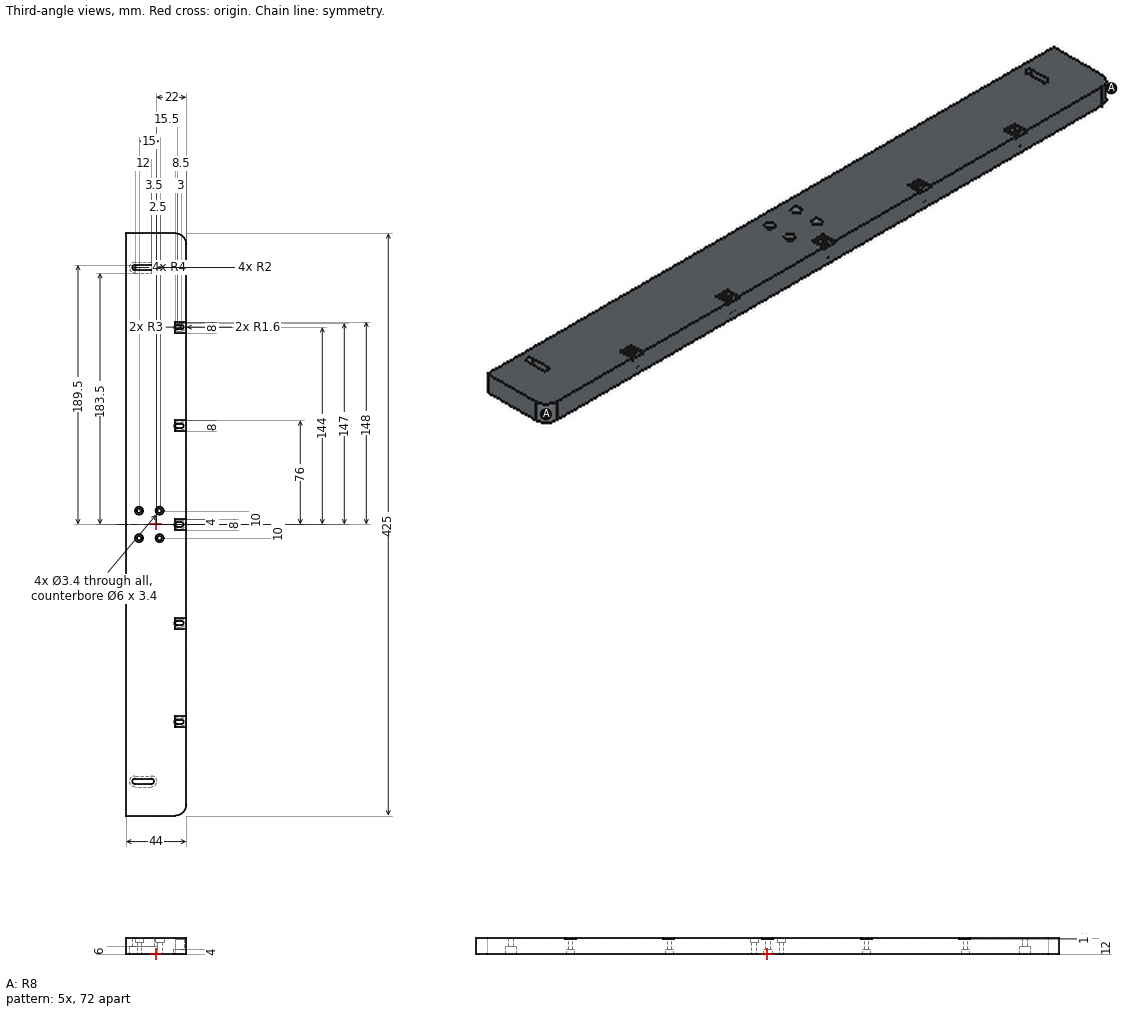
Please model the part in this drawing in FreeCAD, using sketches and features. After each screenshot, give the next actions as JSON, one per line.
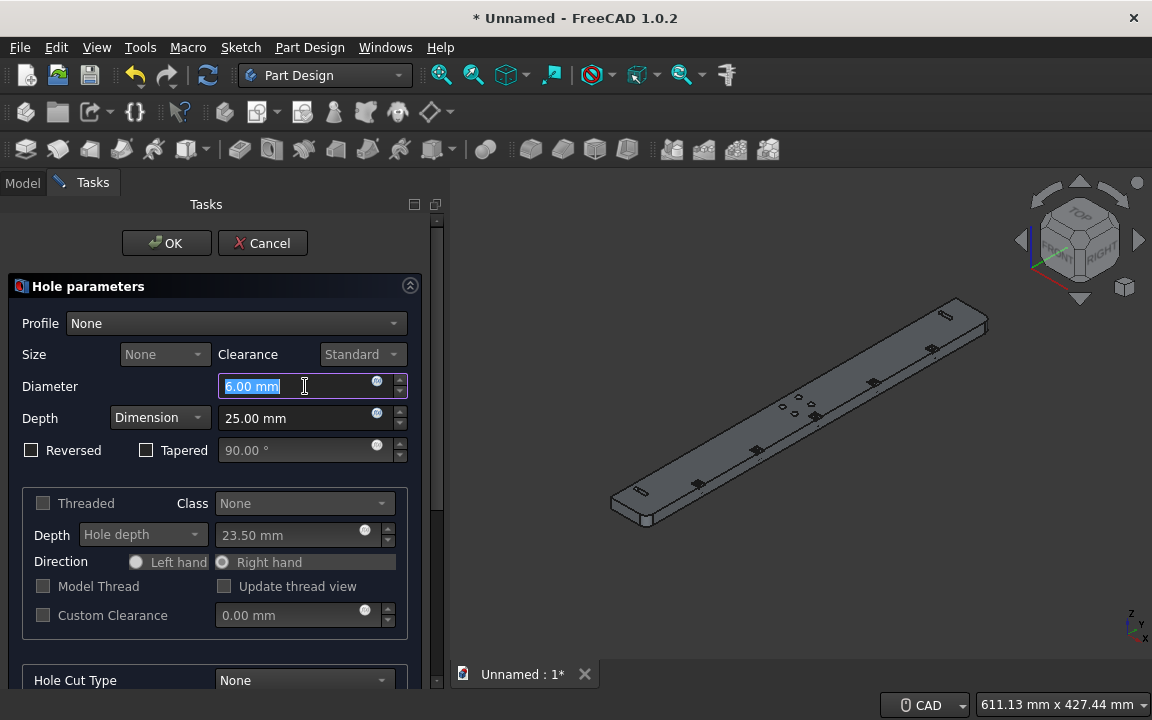
{"action": "type", "text": "3.4"}
{"action": "key", "text": "Tab"}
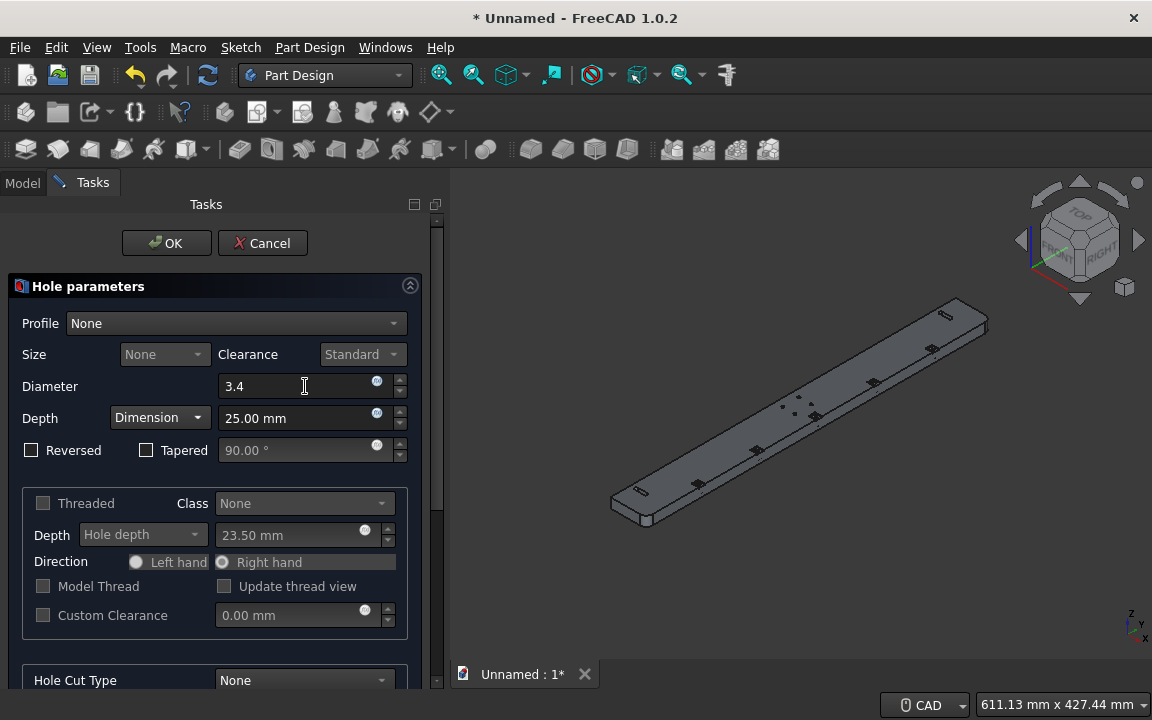
{"action": "left_click", "coordinate": [161, 418]}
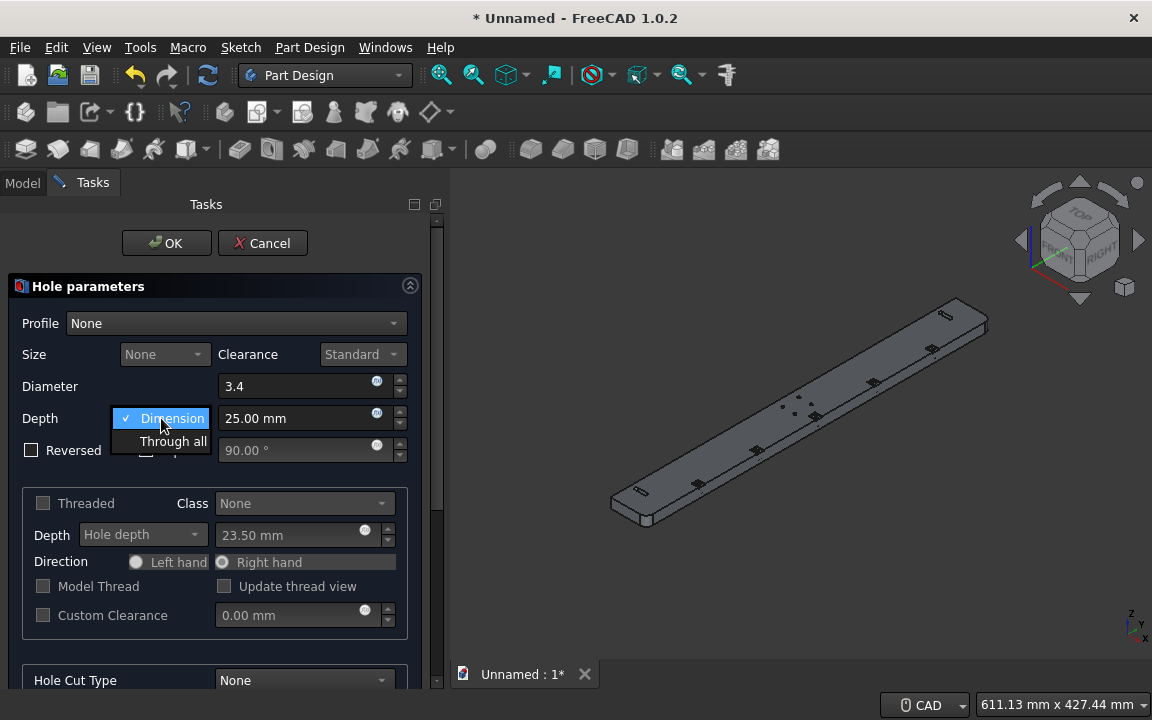
{"action": "left_click", "coordinate": [160, 442]}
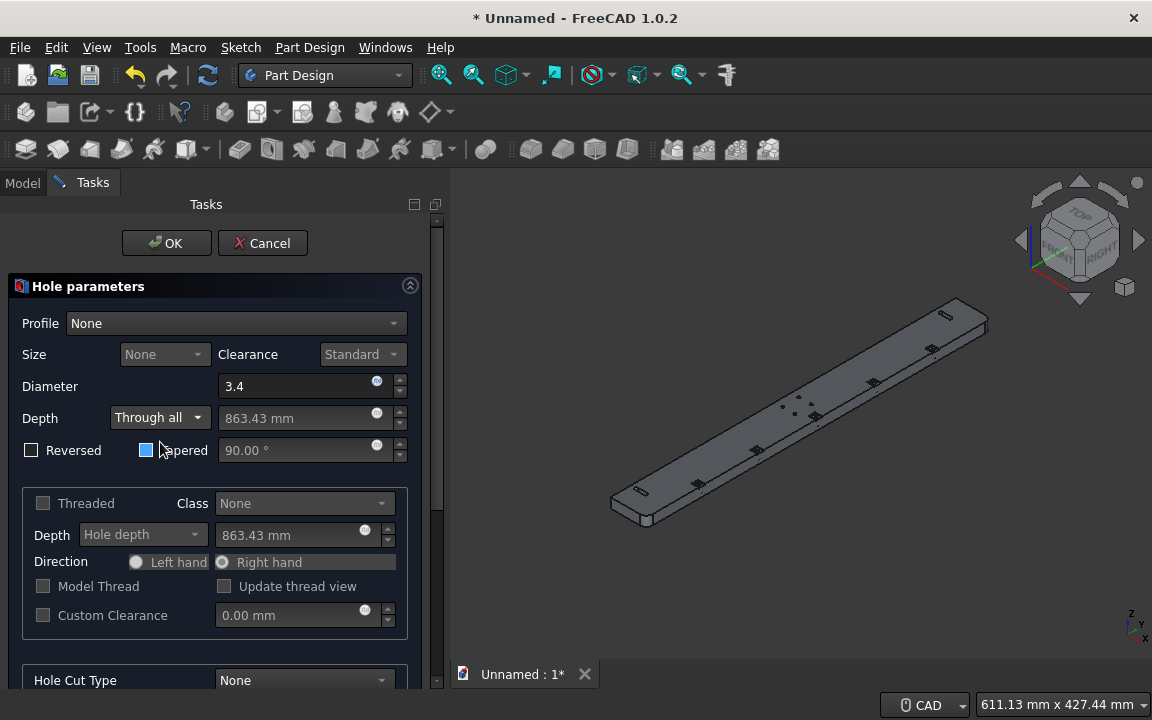
{"action": "scroll", "coordinate": [437, 451], "scroll_direction": "down", "scroll_amount": 2}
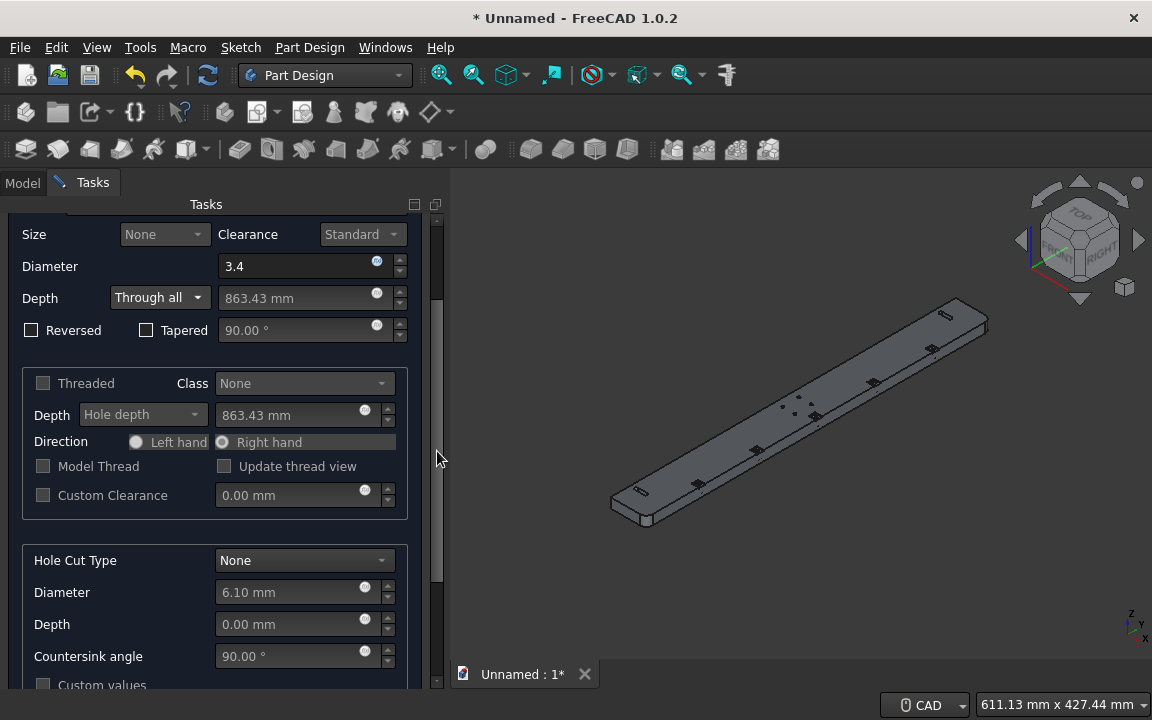
{"action": "left_click", "coordinate": [306, 560]}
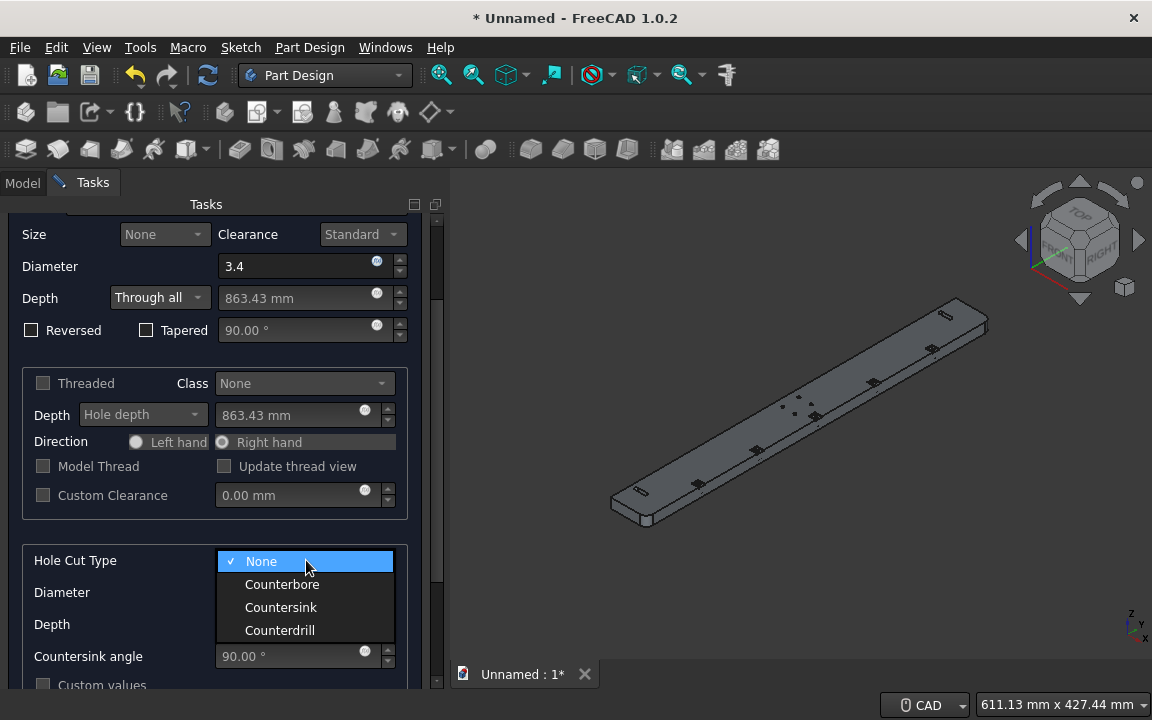
{"action": "left_click", "coordinate": [304, 584]}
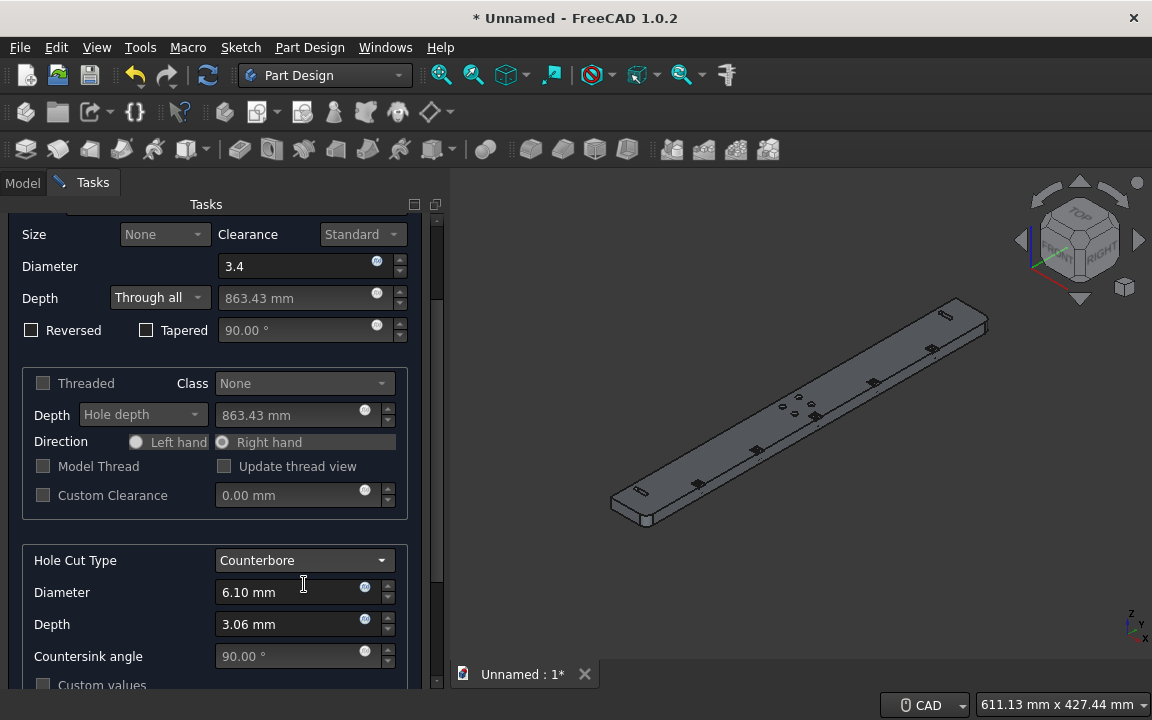
{"action": "triple_click", "coordinate": [298, 592]}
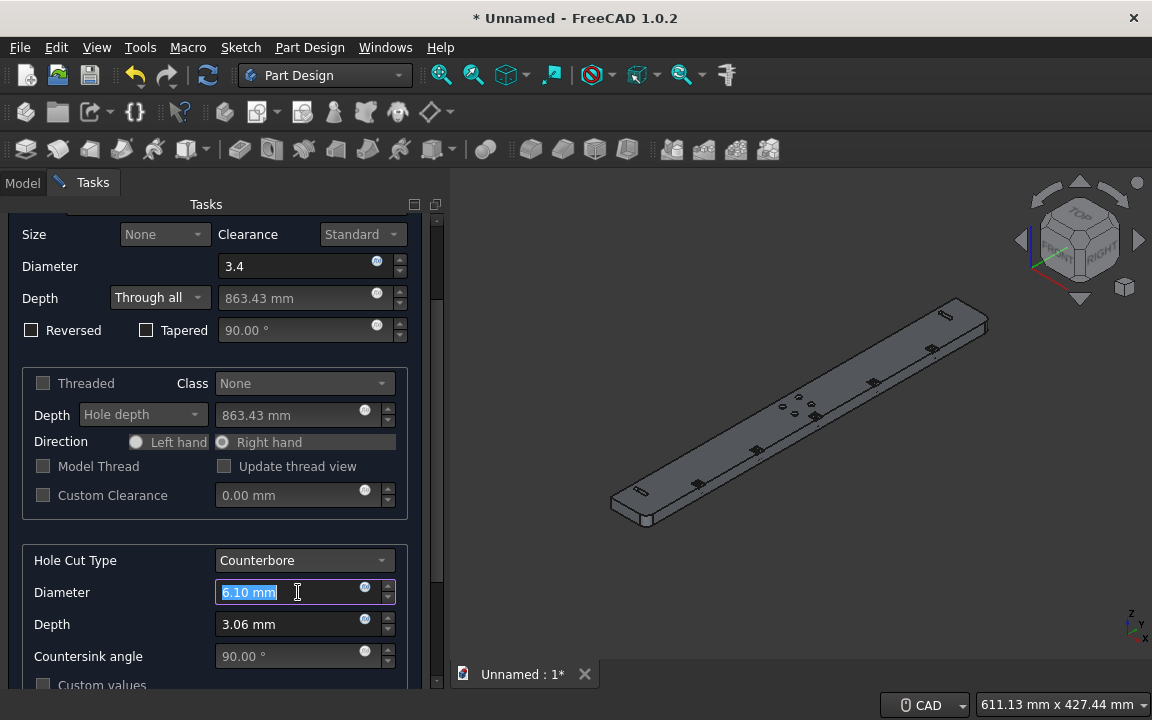
{"action": "type", "text": "6"}
{"action": "key", "text": "Tab"}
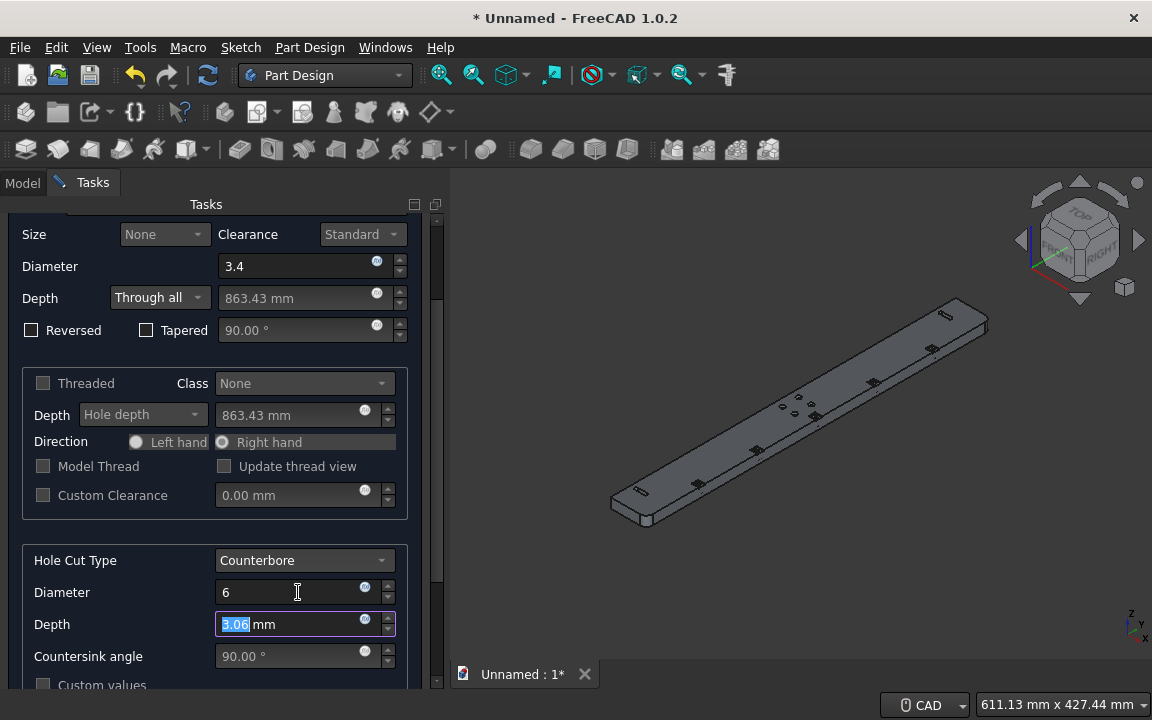
{"action": "type", "text": "3.4"}
{"action": "key", "text": "Tab"}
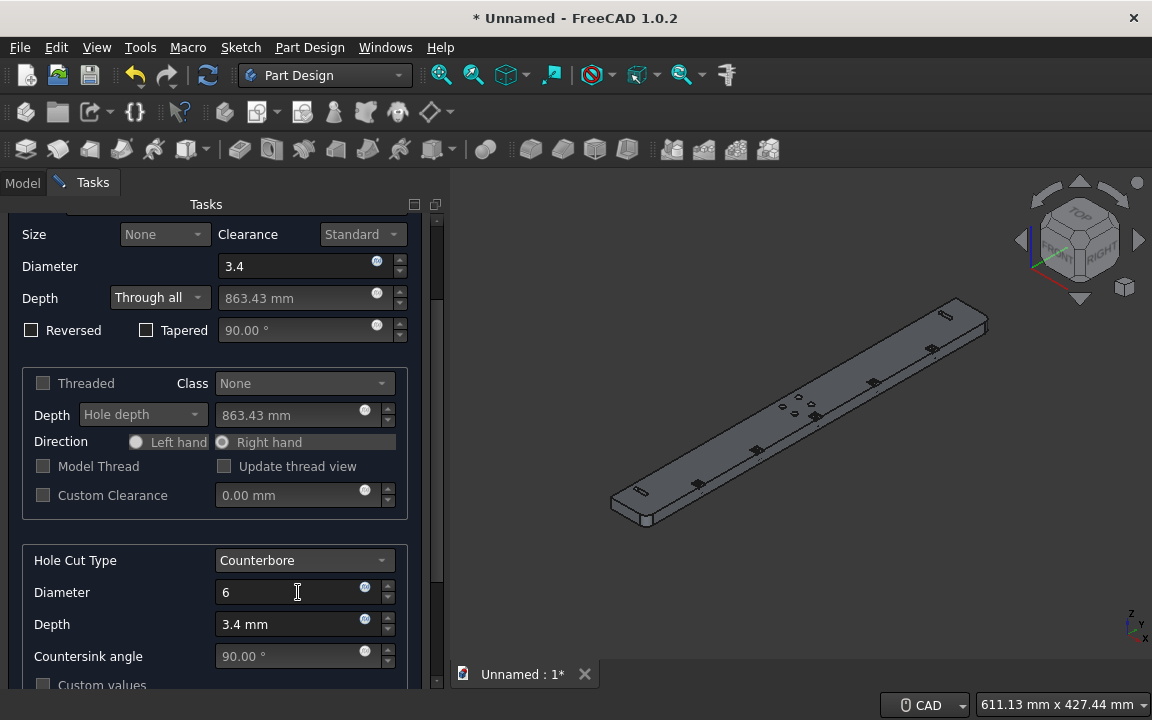
{"action": "scroll", "coordinate": [437, 451], "scroll_direction": "up", "scroll_amount": 3}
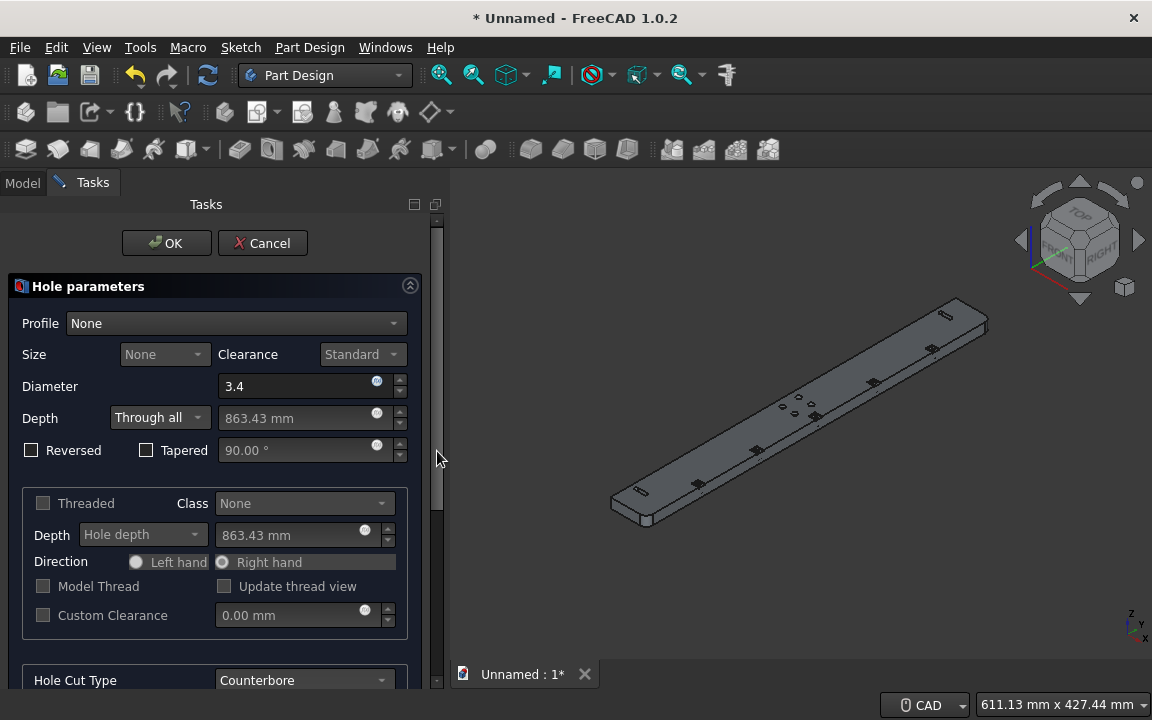
{"action": "left_click", "coordinate": [167, 243]}